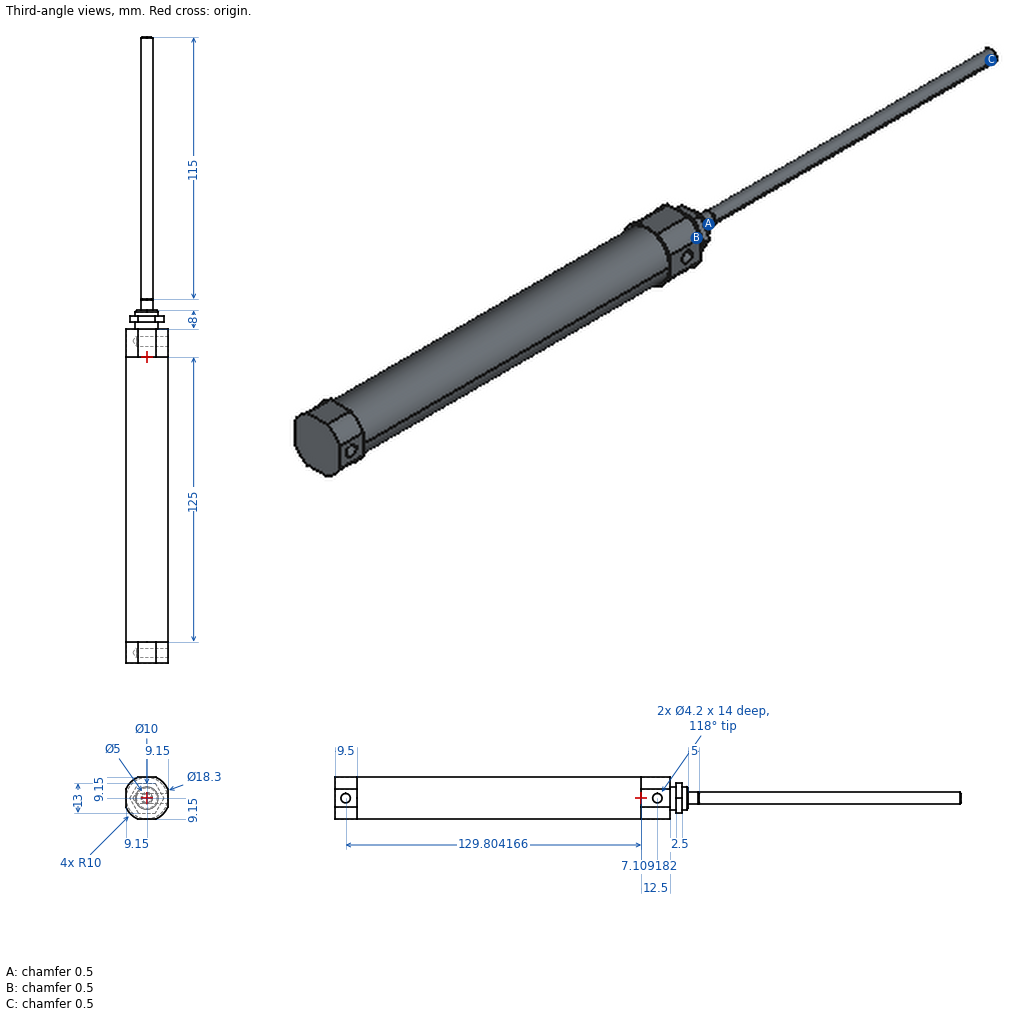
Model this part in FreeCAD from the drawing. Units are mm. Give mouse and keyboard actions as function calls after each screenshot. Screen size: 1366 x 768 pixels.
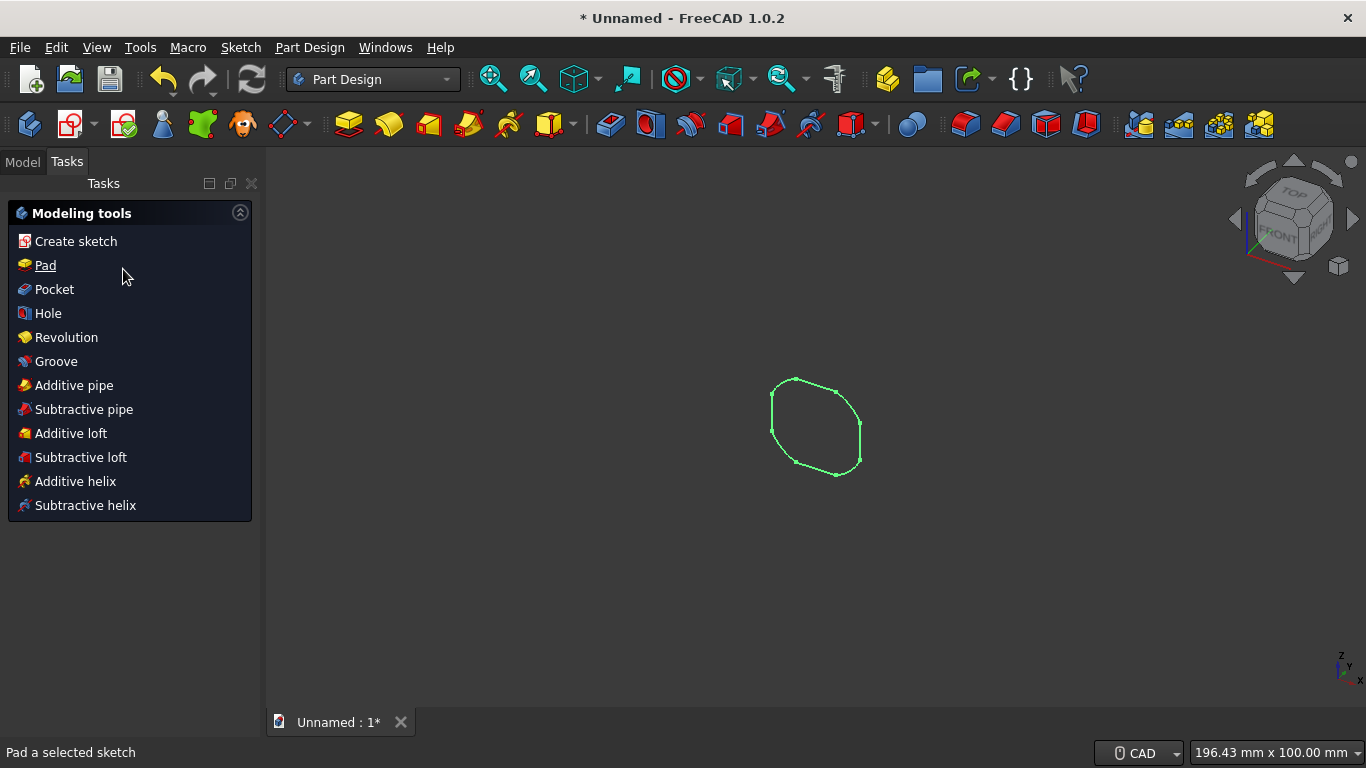
click(350, 124)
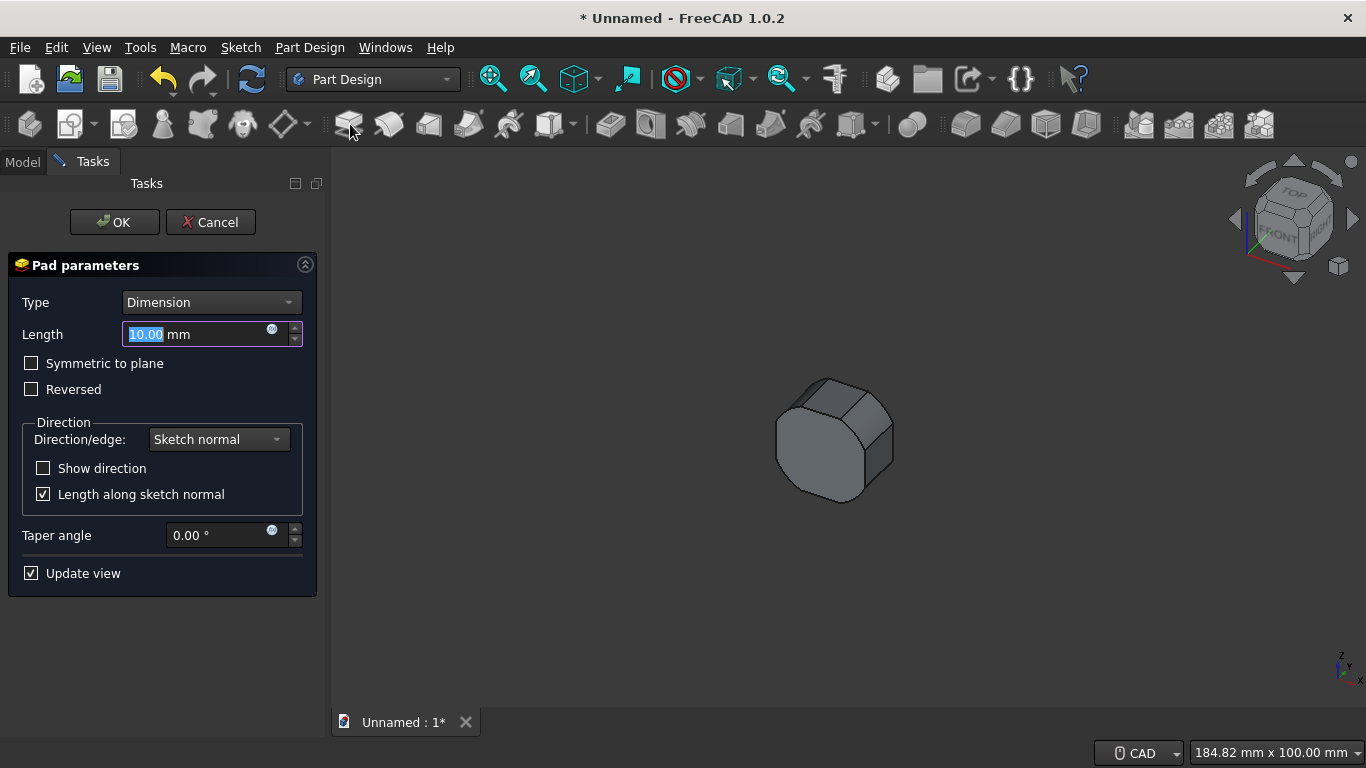
text(12.5)
key(Tab)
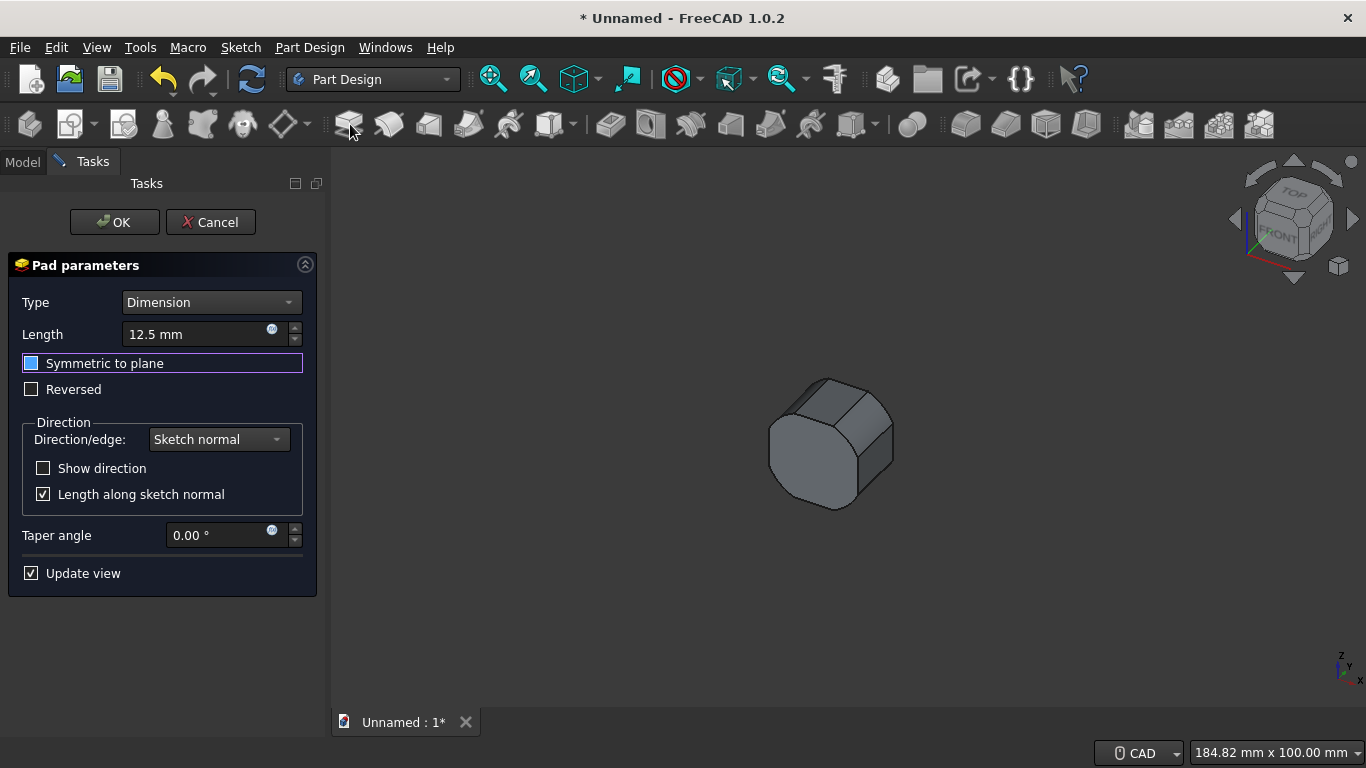
click(30, 389)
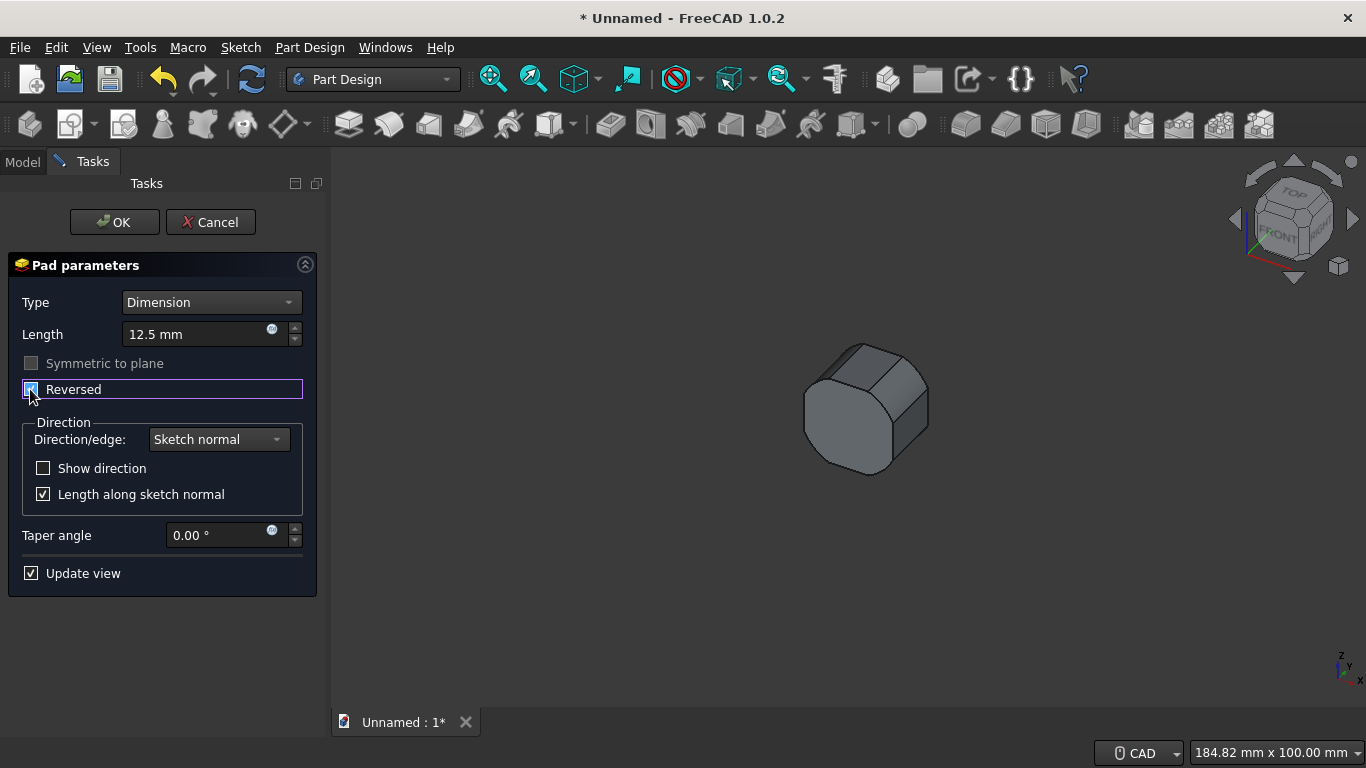
click(115, 222)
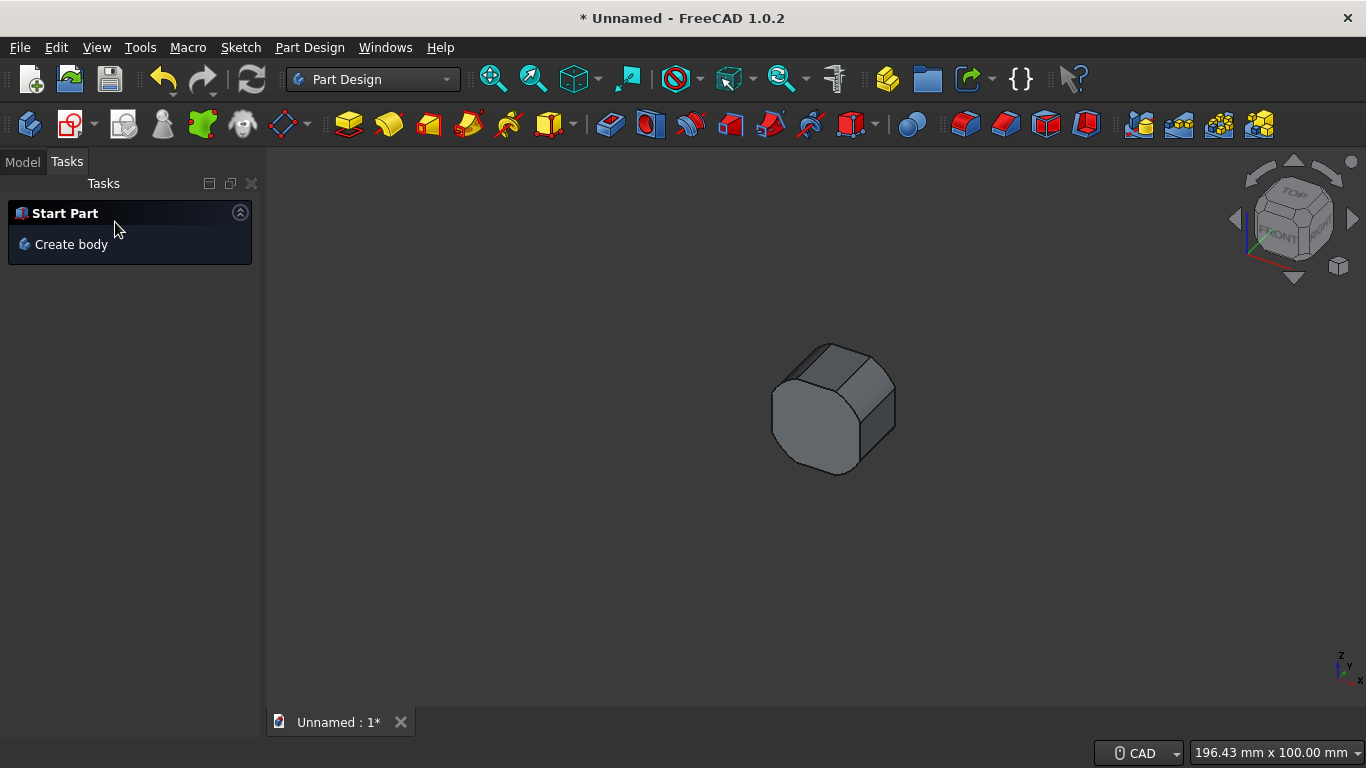
key(v)
key(f)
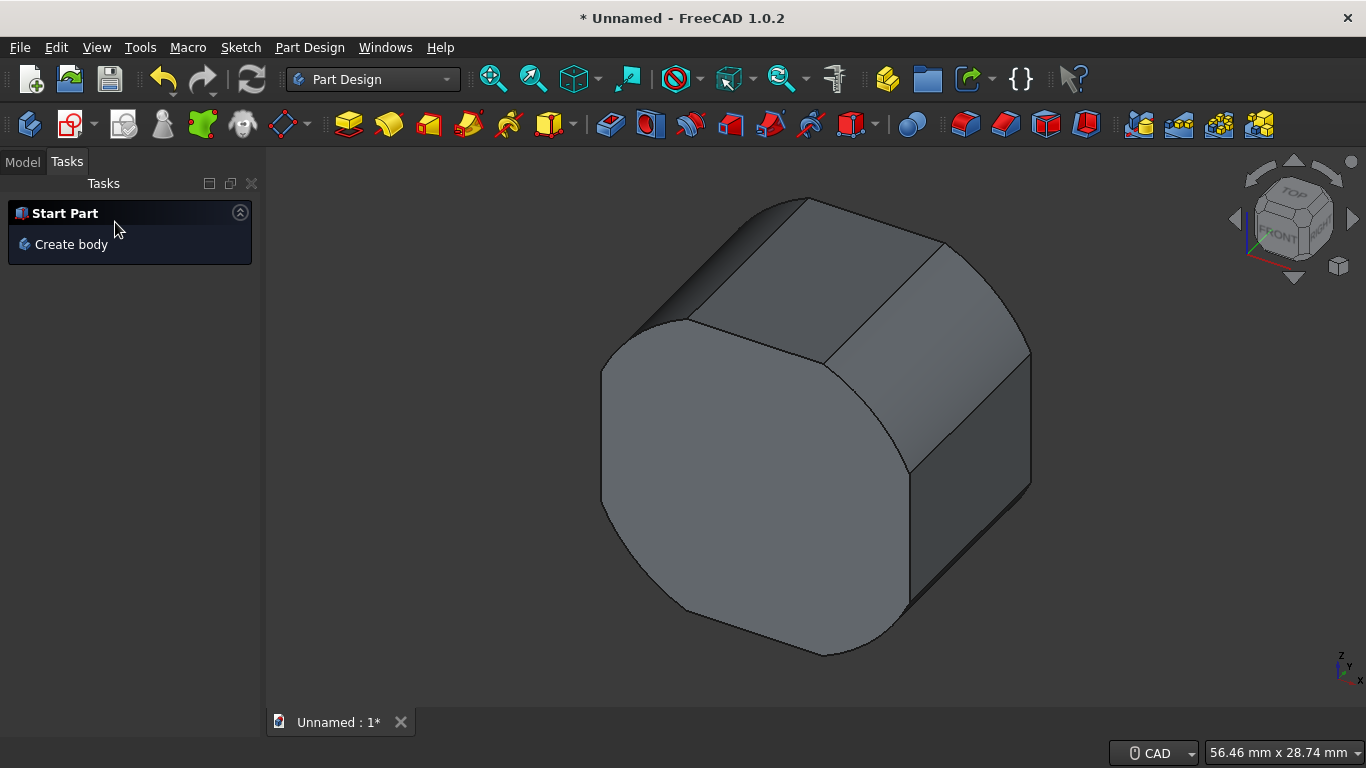
click(755, 486)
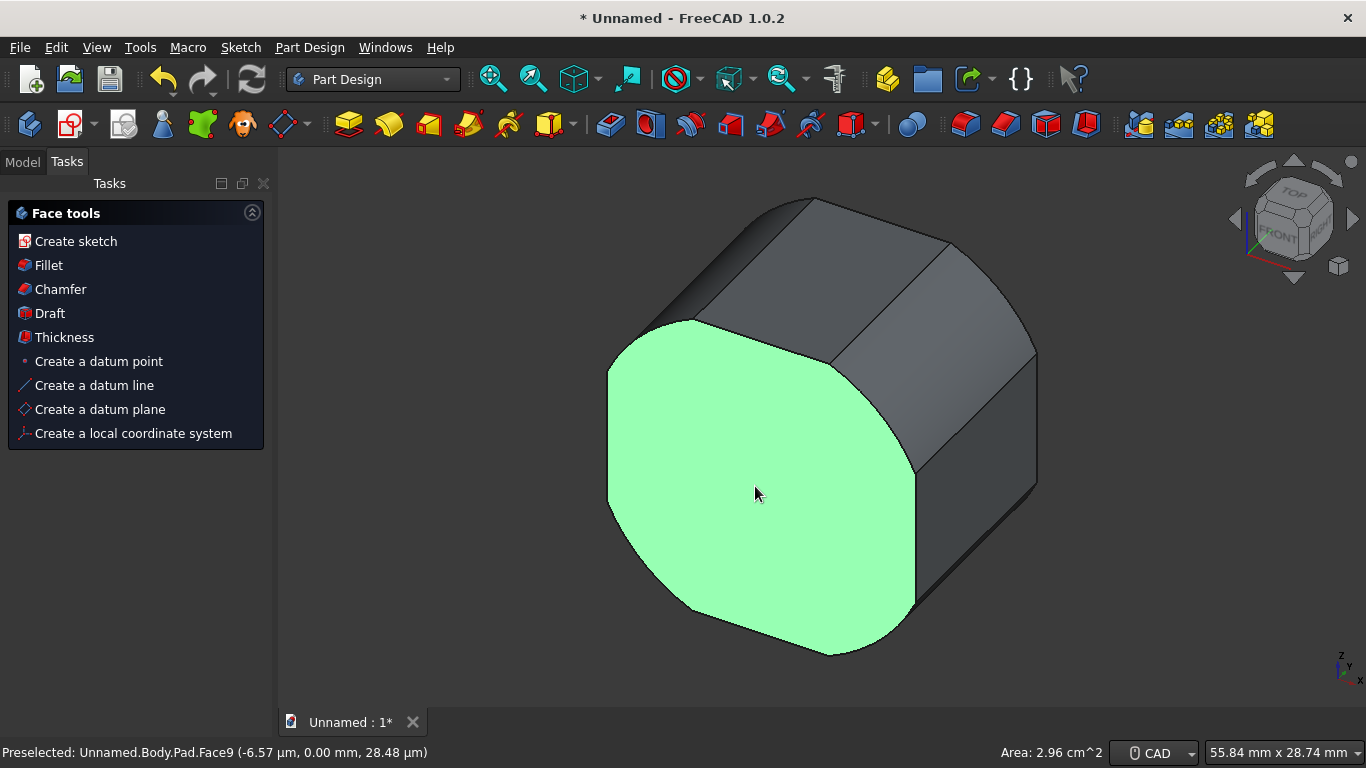
click(70, 124)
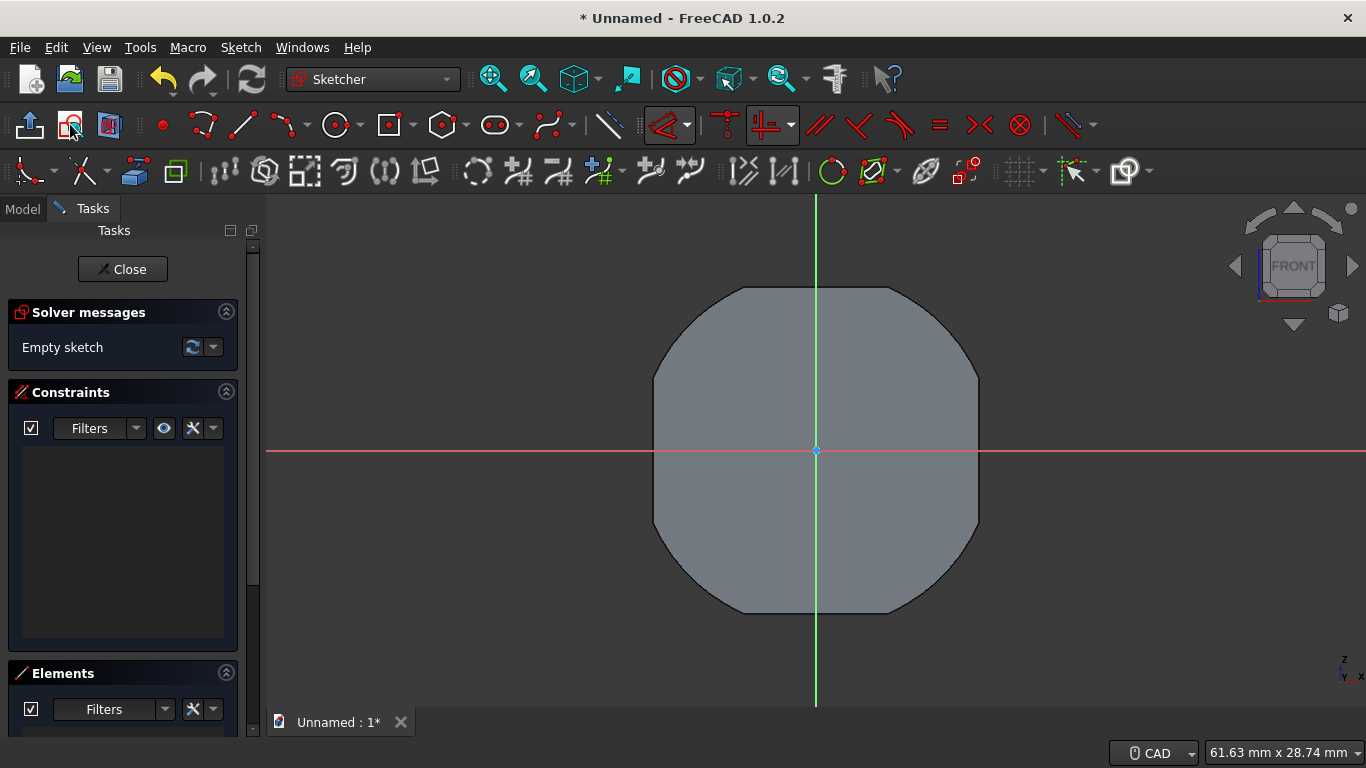
key(g)
key(c)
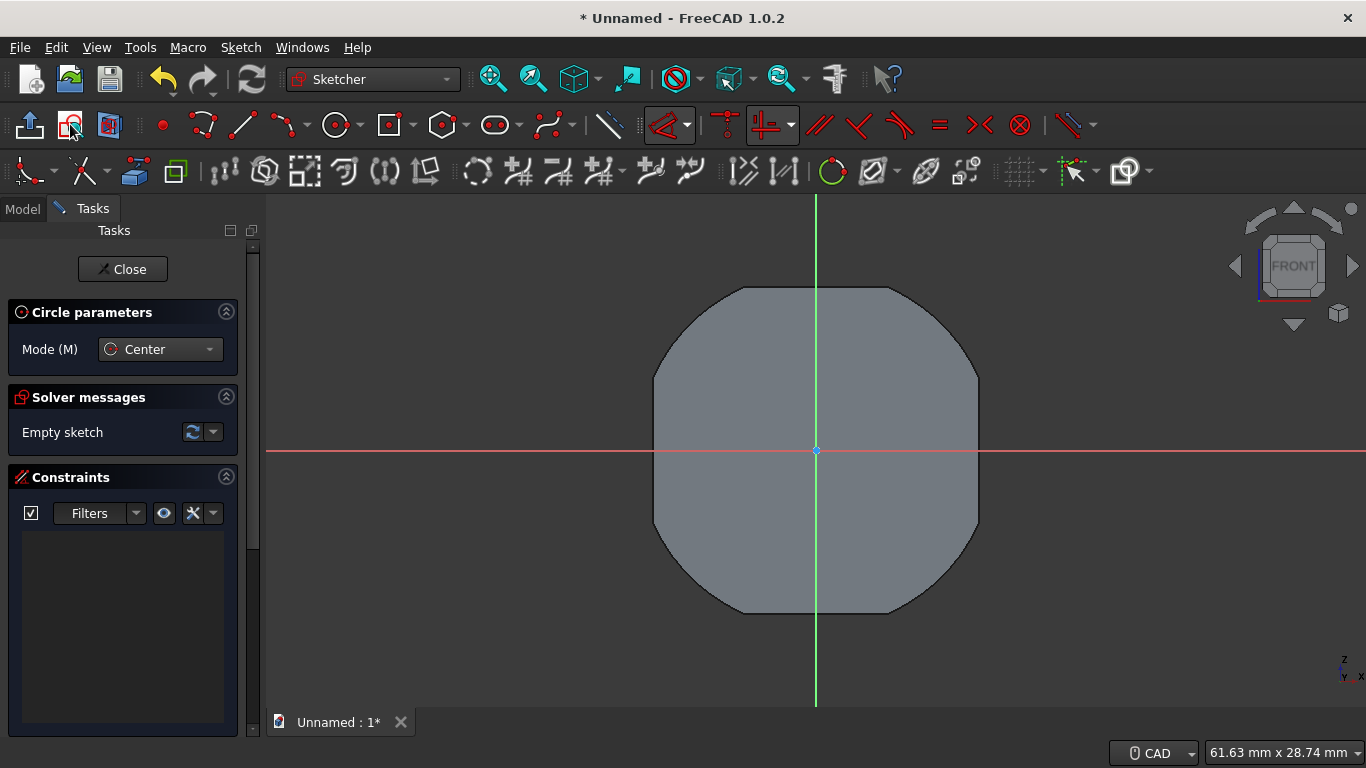
click(816, 451)
click(931, 335)
key(Escape)